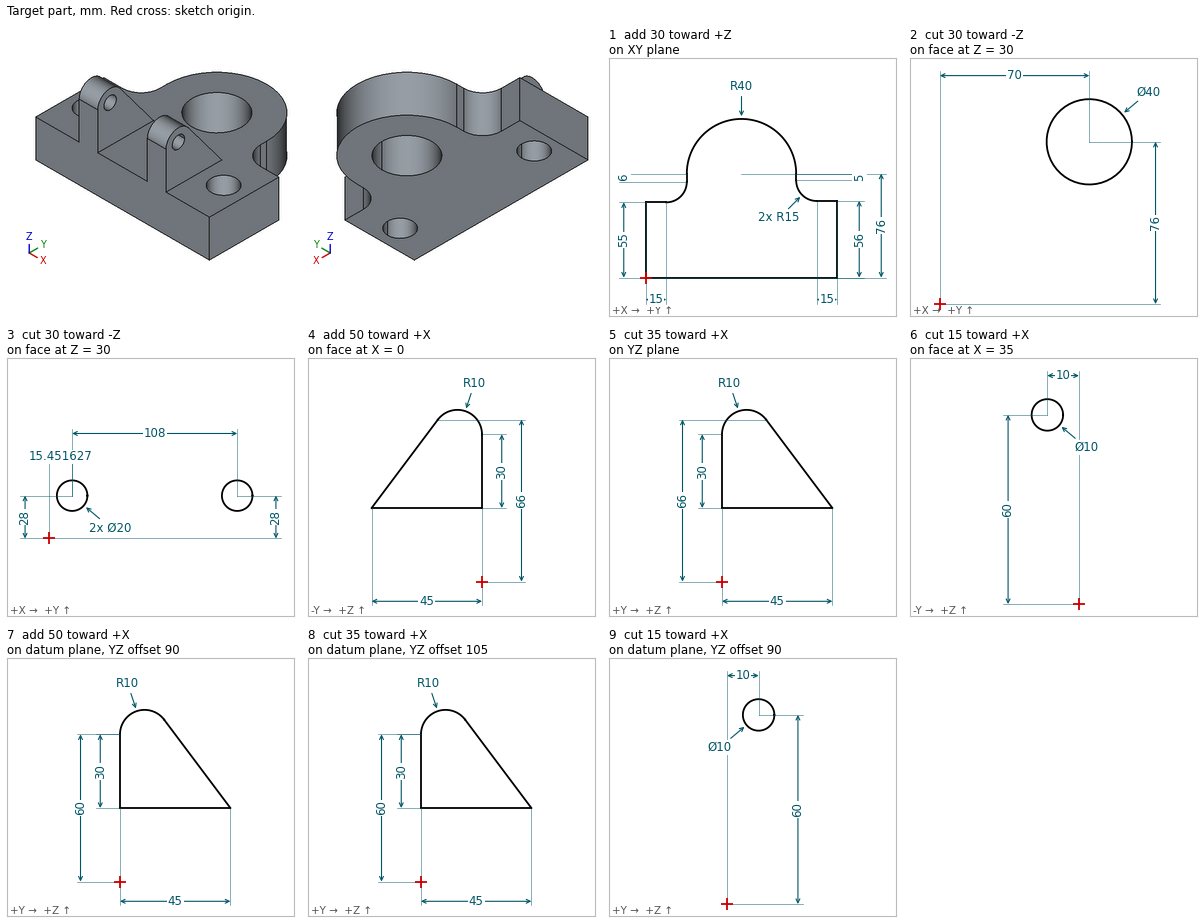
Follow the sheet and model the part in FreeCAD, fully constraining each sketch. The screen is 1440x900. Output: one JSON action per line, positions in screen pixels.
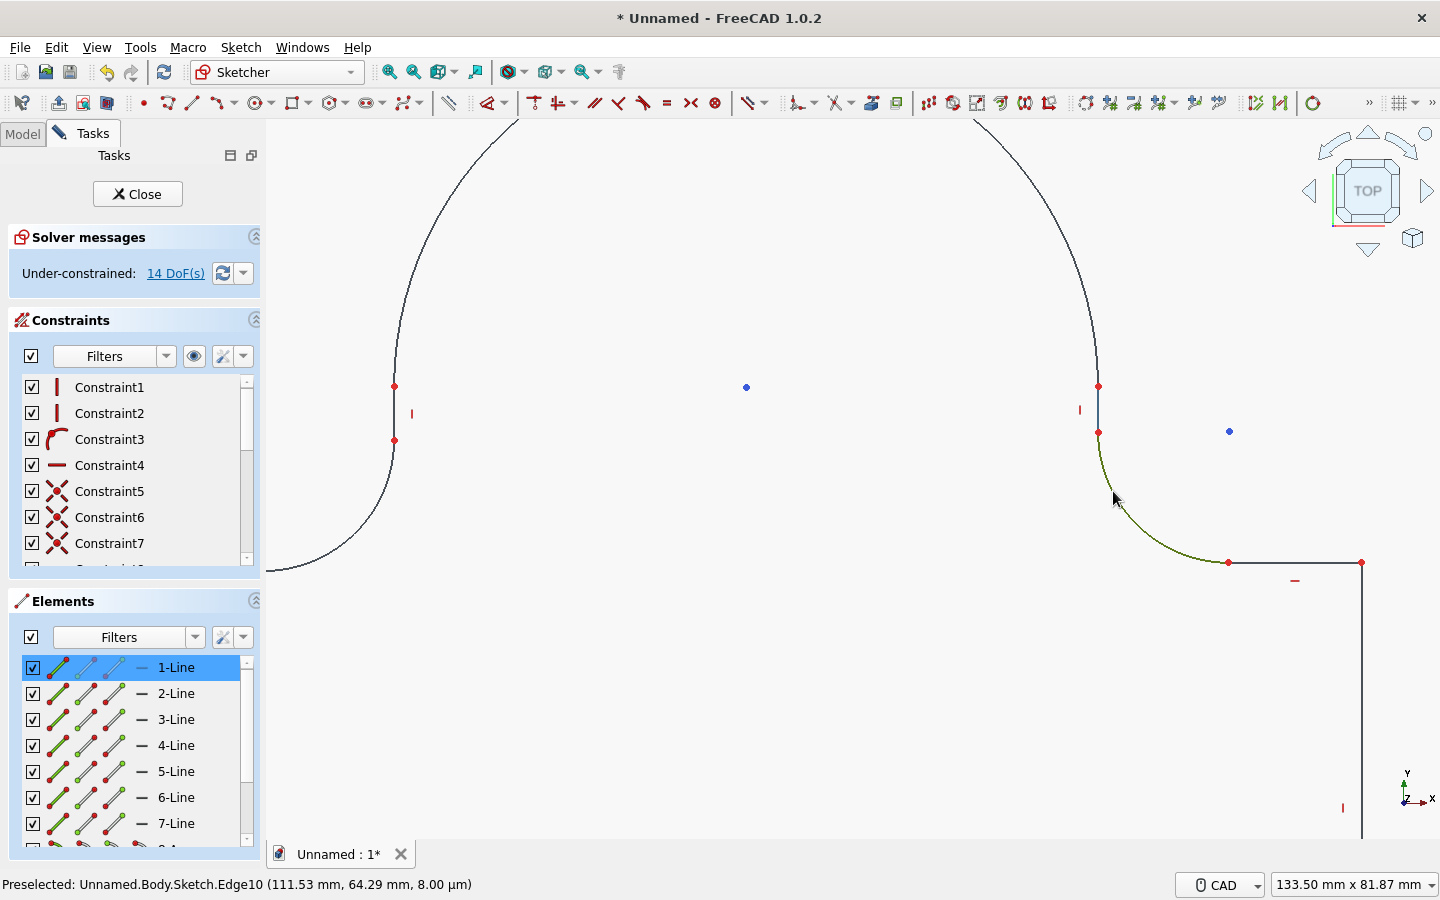
{"action": "key", "text": "t"}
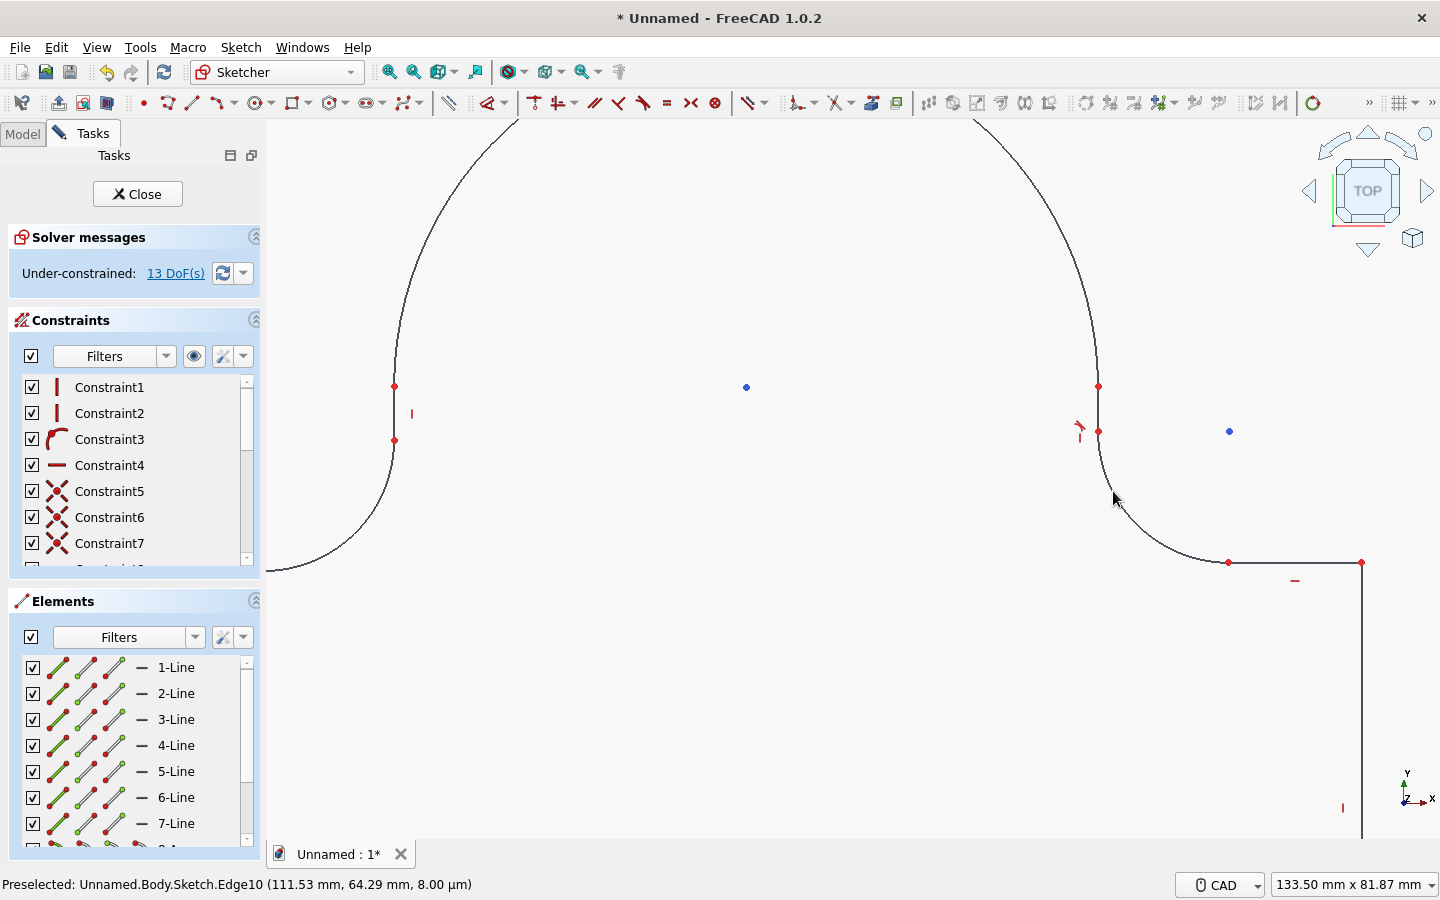
{"action": "left_click", "coordinate": [394, 402]}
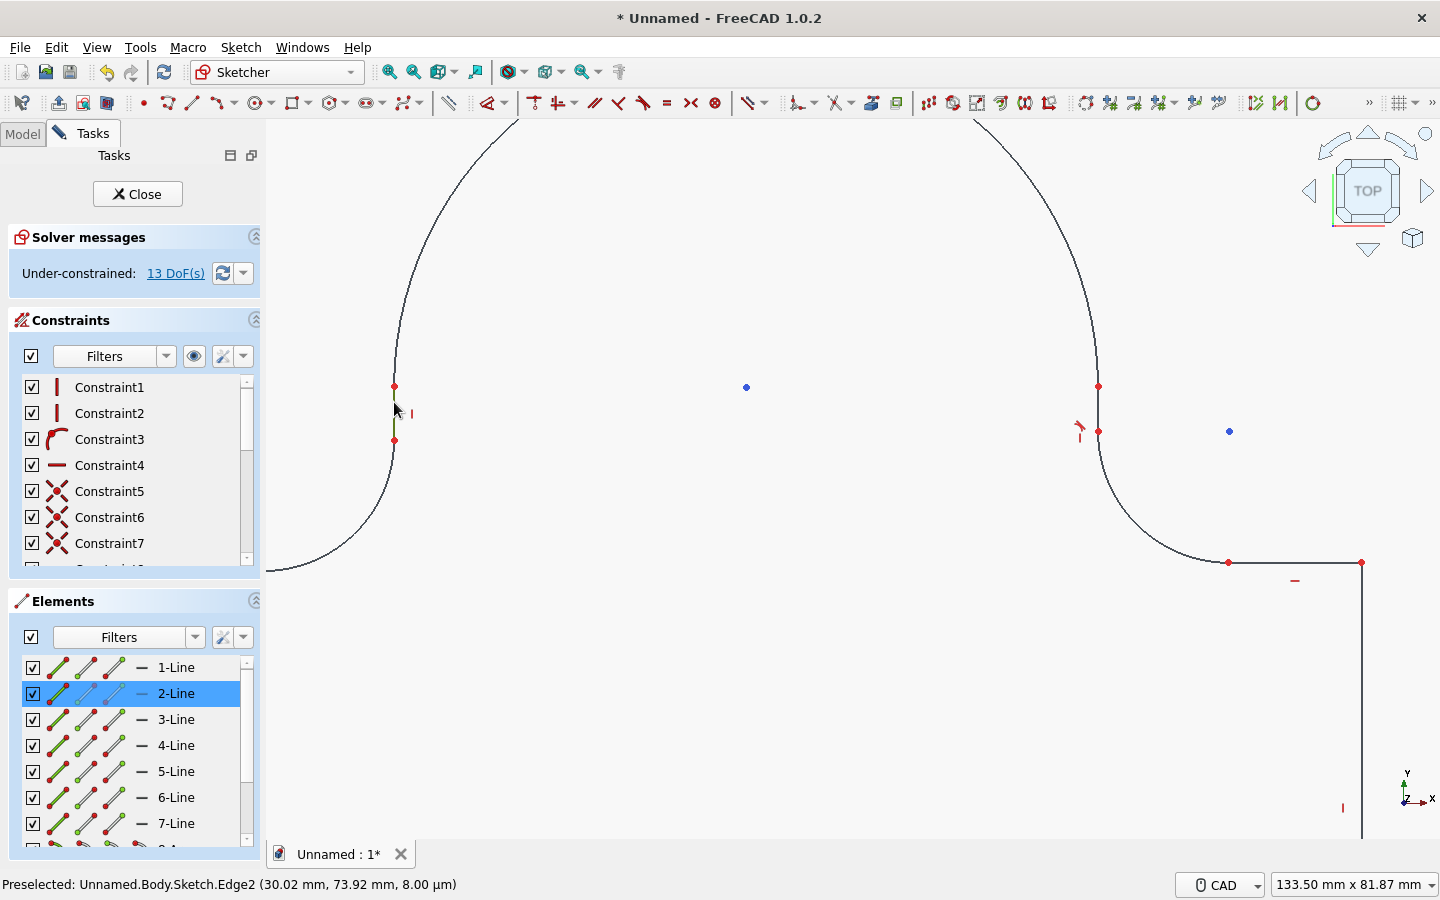
{"action": "left_click", "coordinate": [321, 558]}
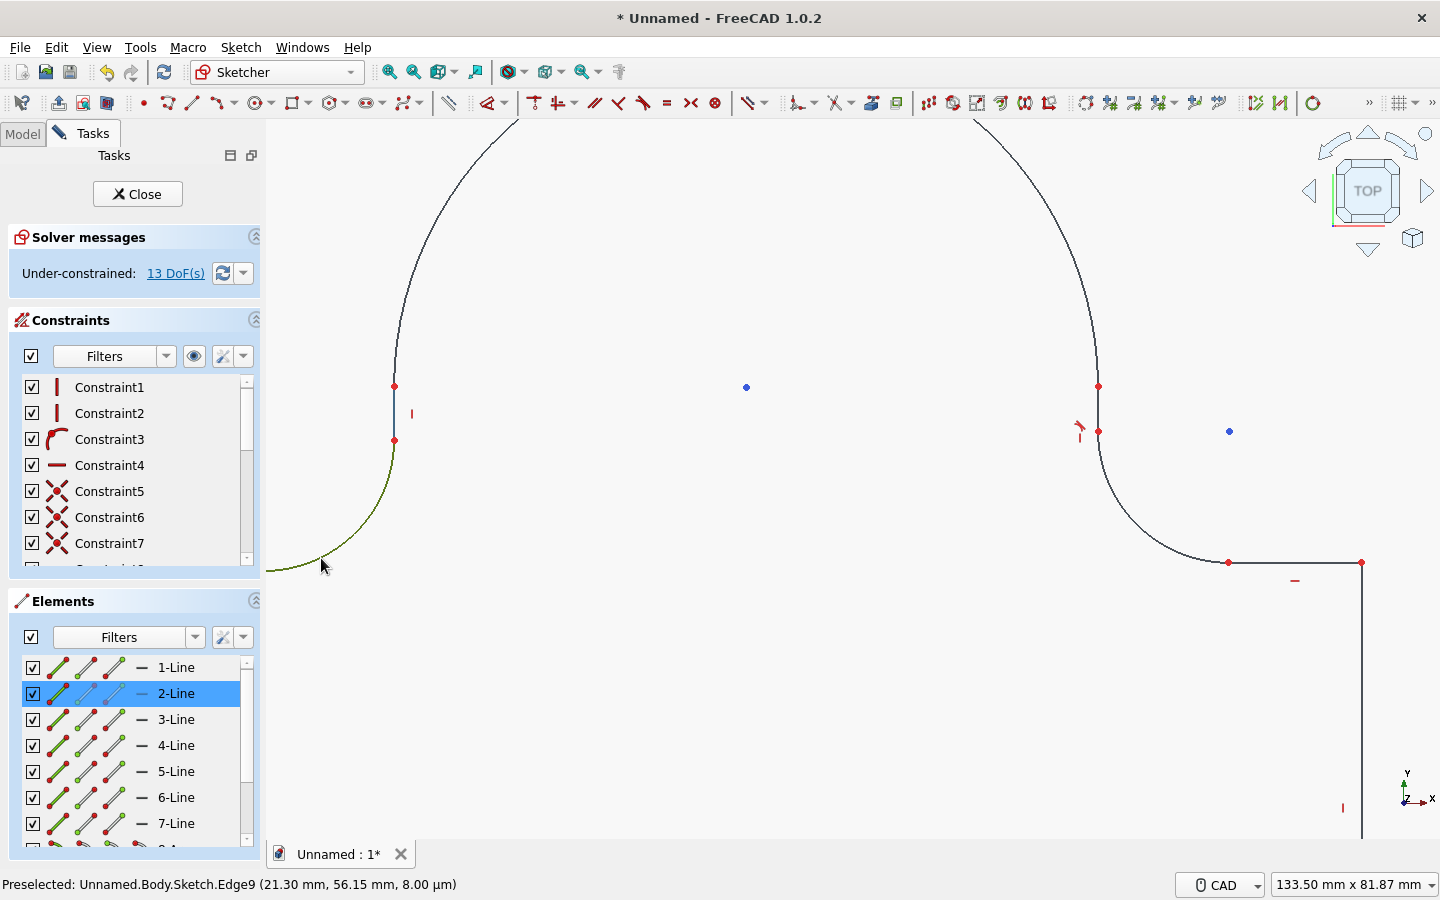
{"action": "key", "text": "t"}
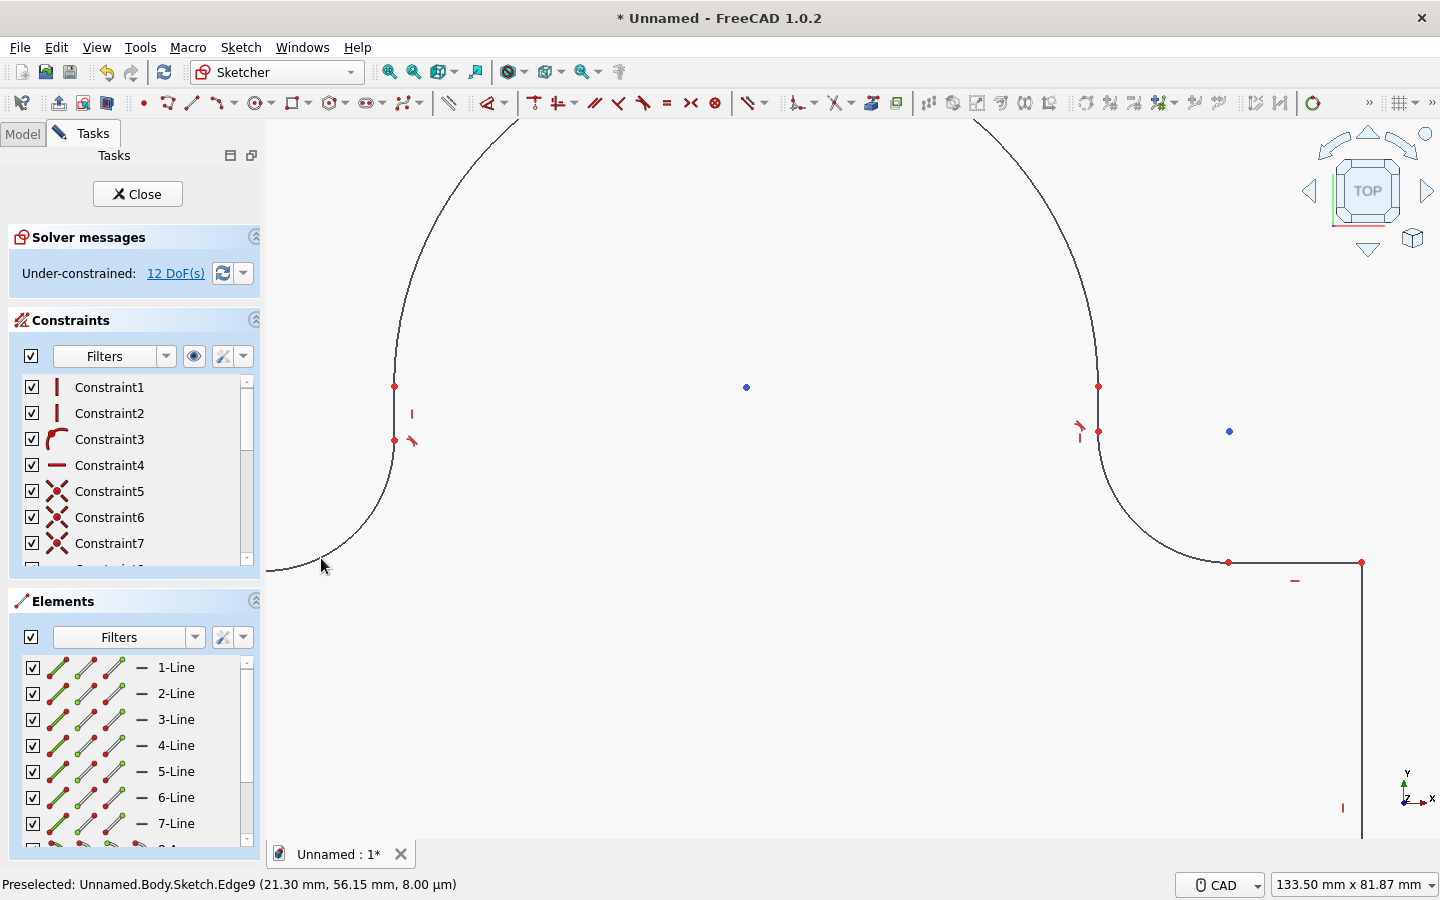
{"action": "scroll", "coordinate": [816, 427], "scroll_direction": "down", "scroll_amount": 4}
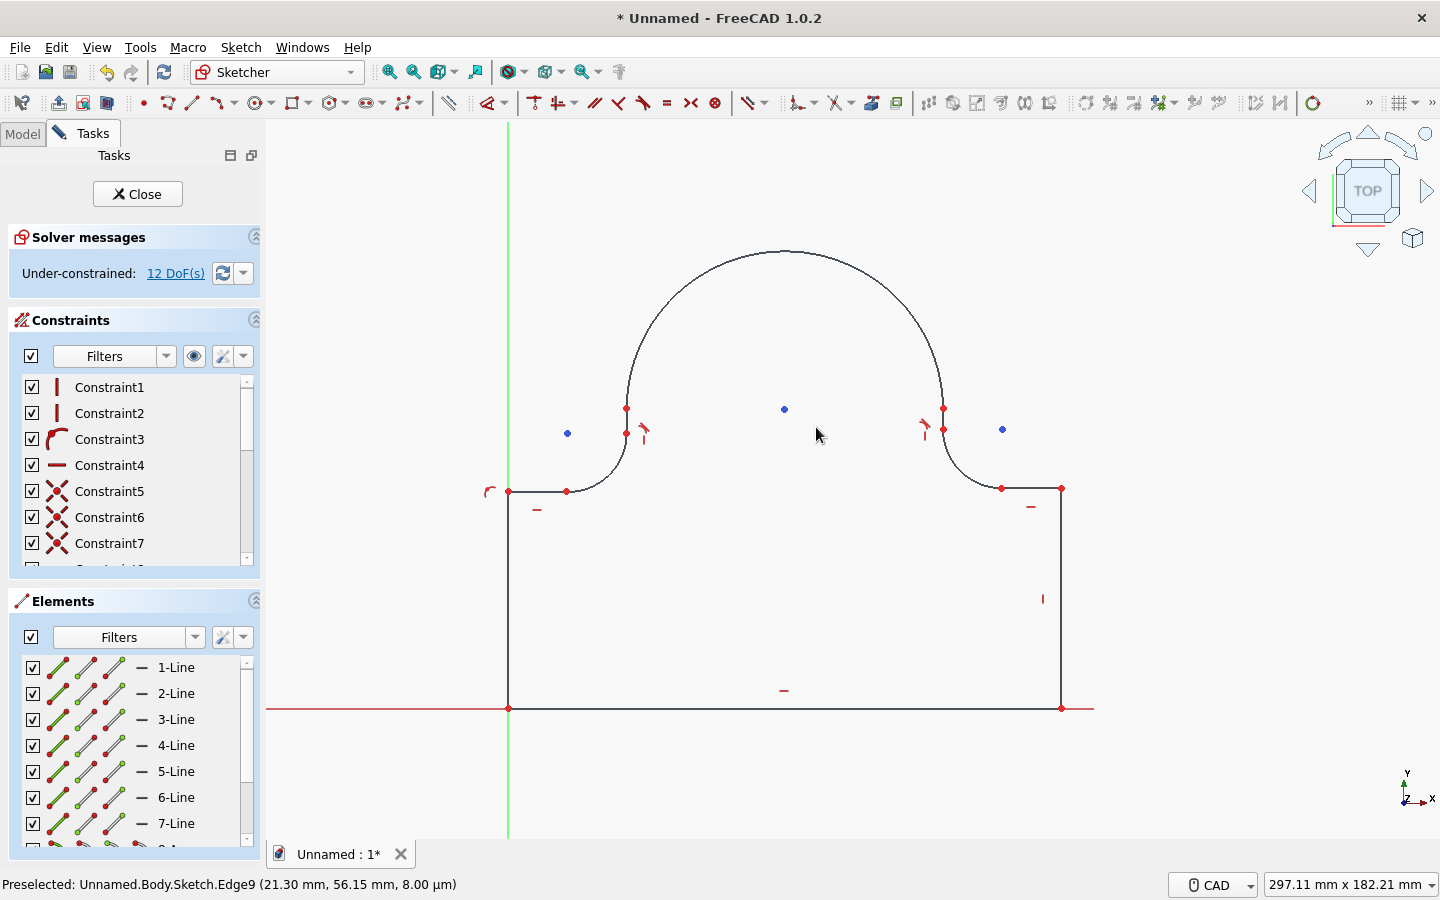
{"action": "left_click", "coordinate": [549, 492]}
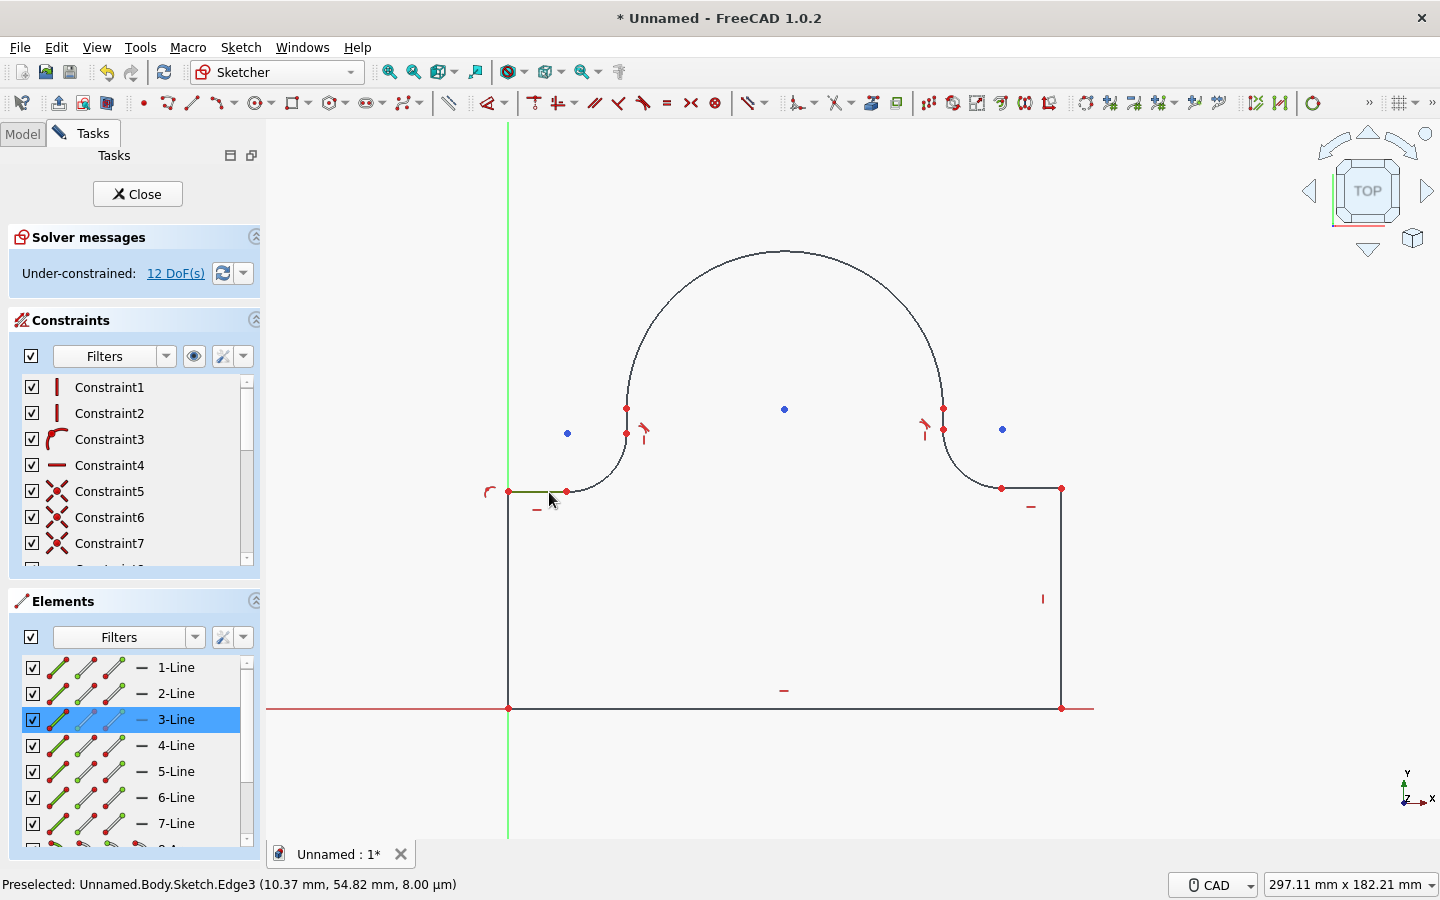
{"action": "left_click", "coordinate": [594, 486]}